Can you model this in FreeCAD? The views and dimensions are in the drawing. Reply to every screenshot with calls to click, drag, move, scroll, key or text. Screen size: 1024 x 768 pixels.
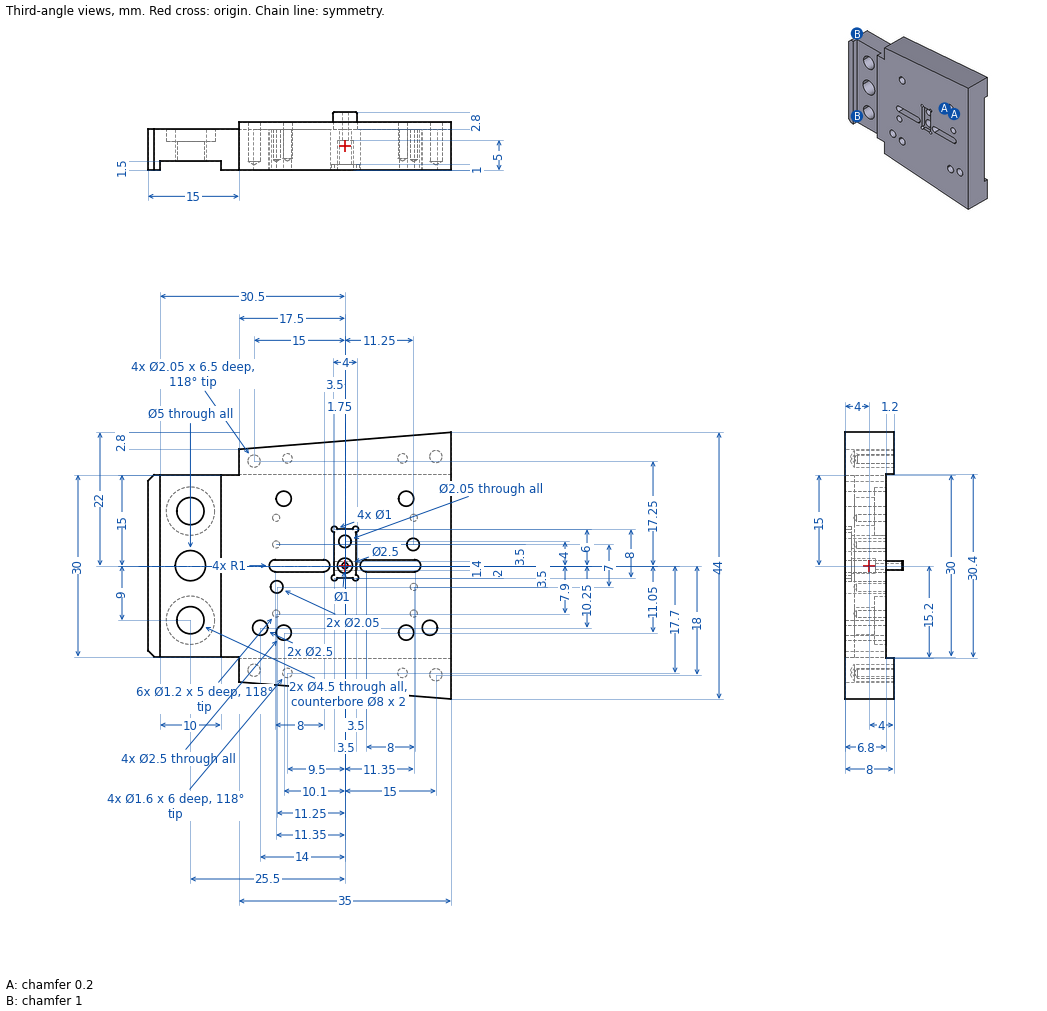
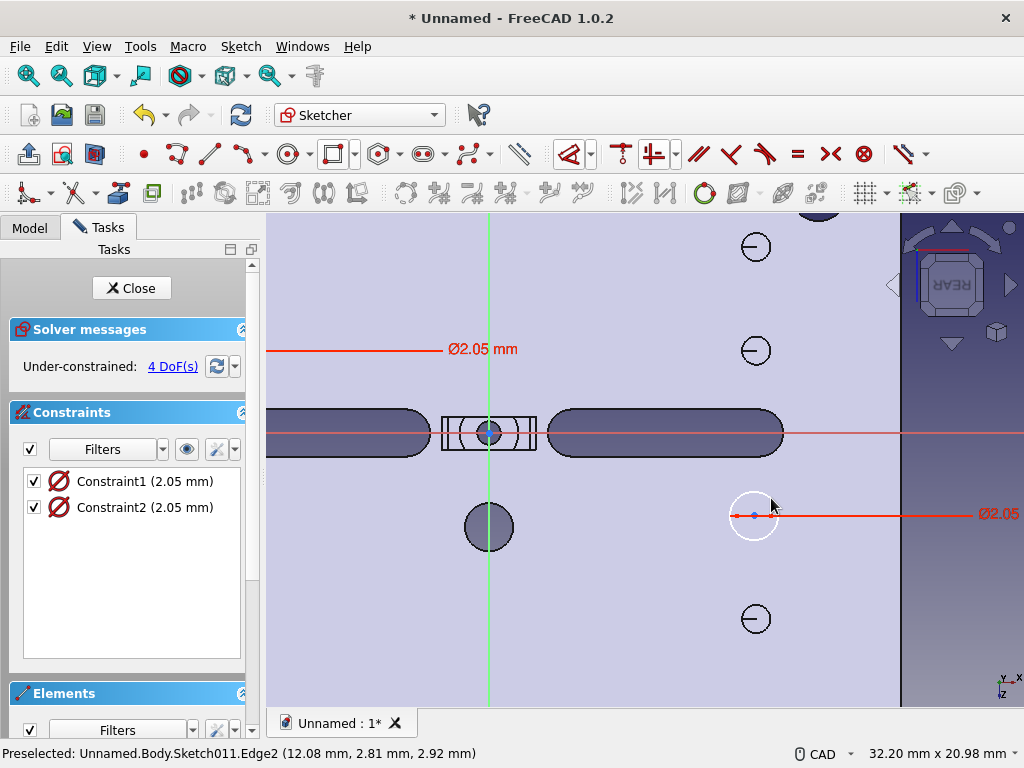
scroll(754, 515, down, 2)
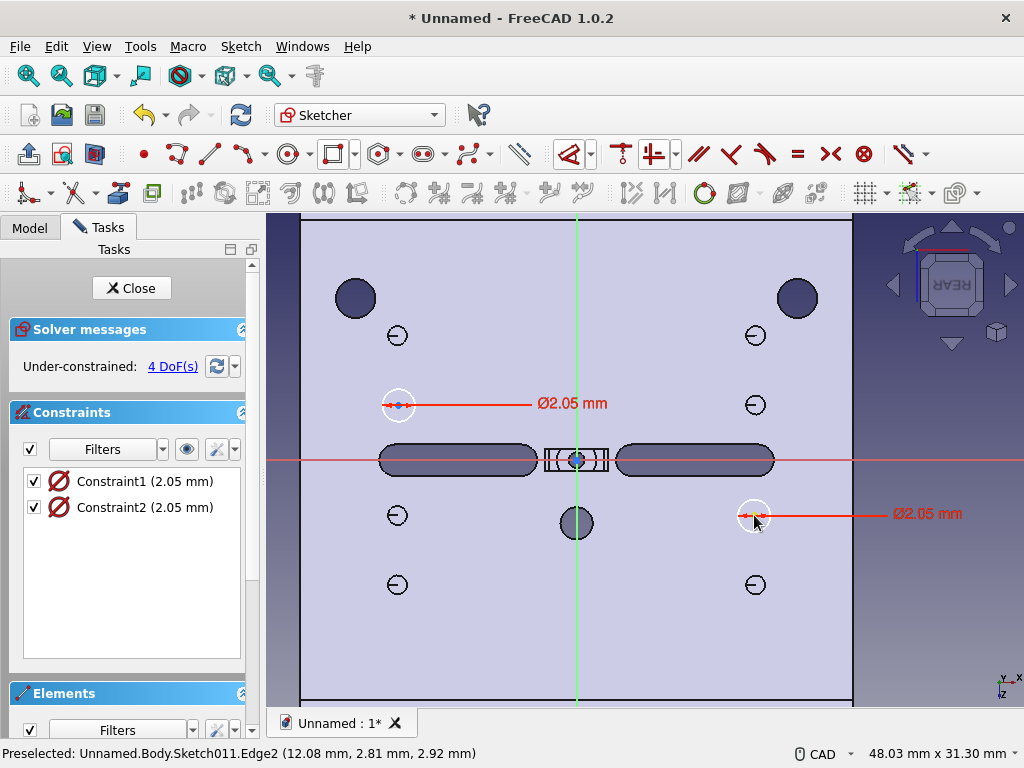
click(399, 405)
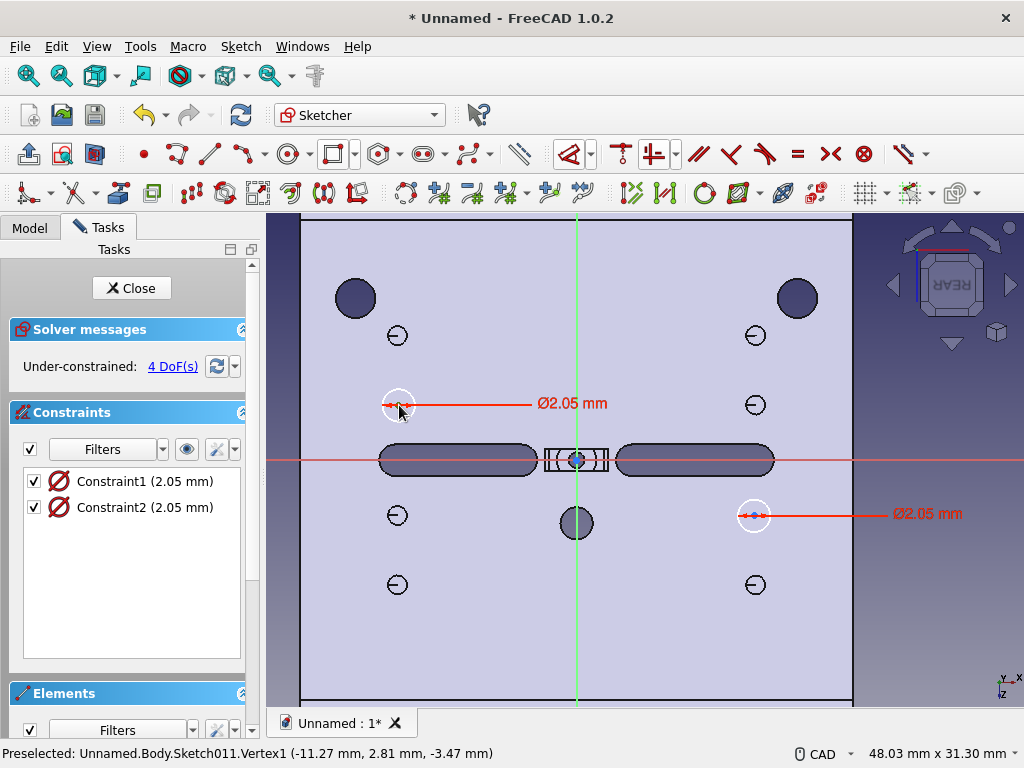
click(754, 516)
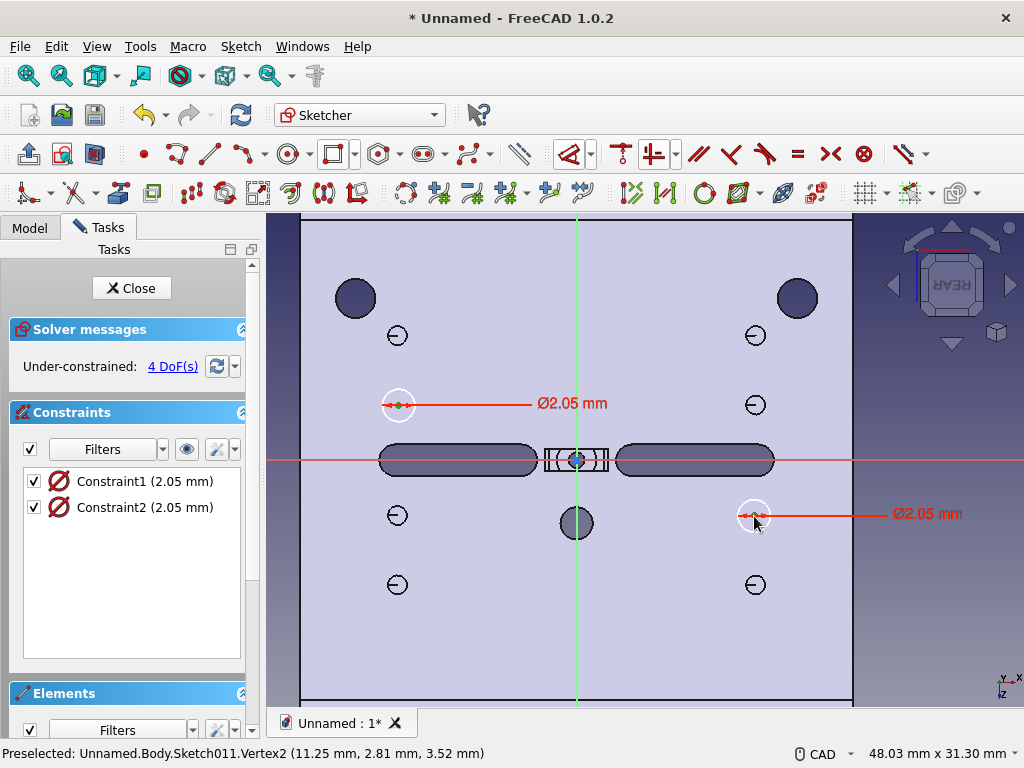
click(590, 154)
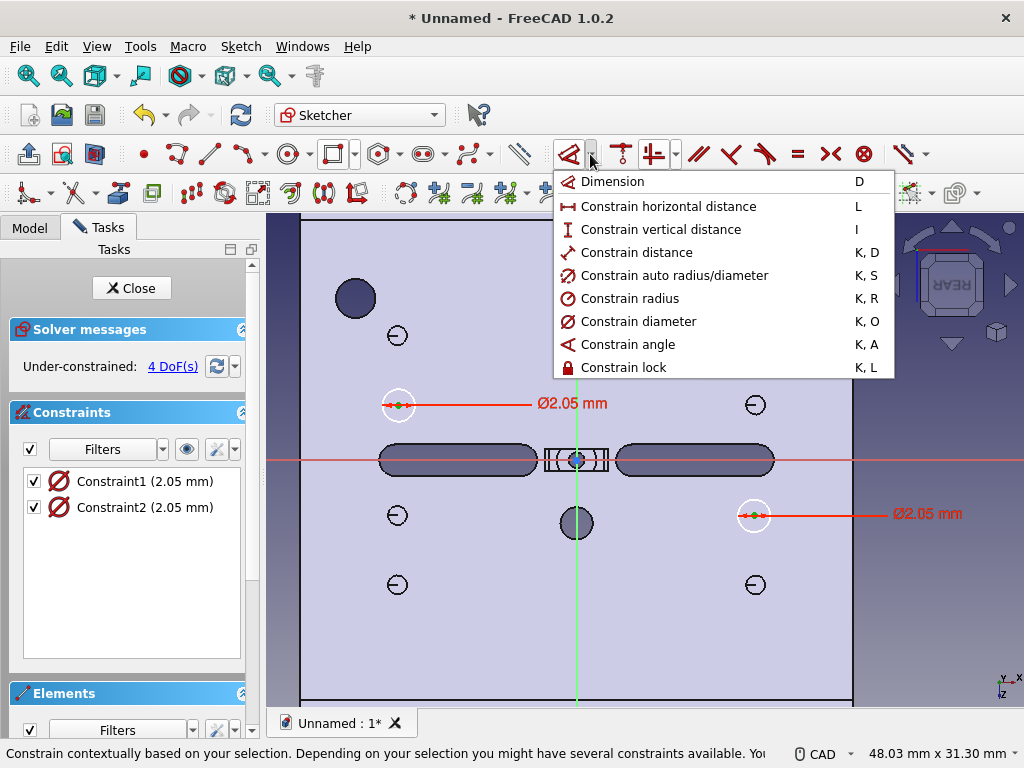
click(724, 230)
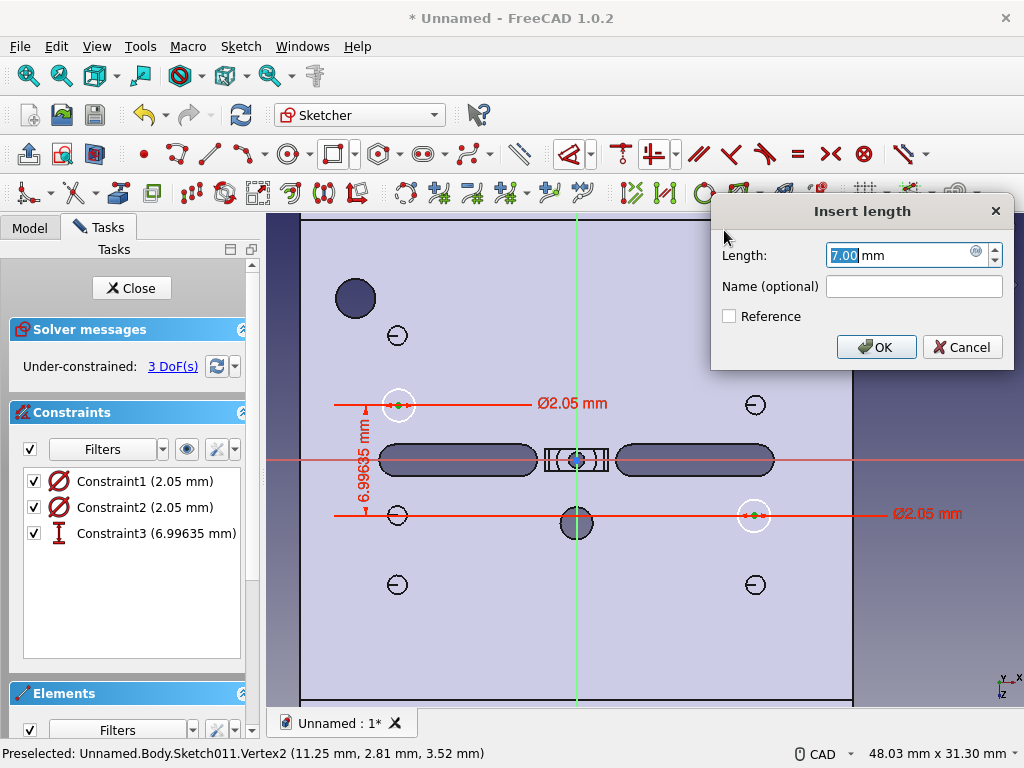
text(7)
key(Return)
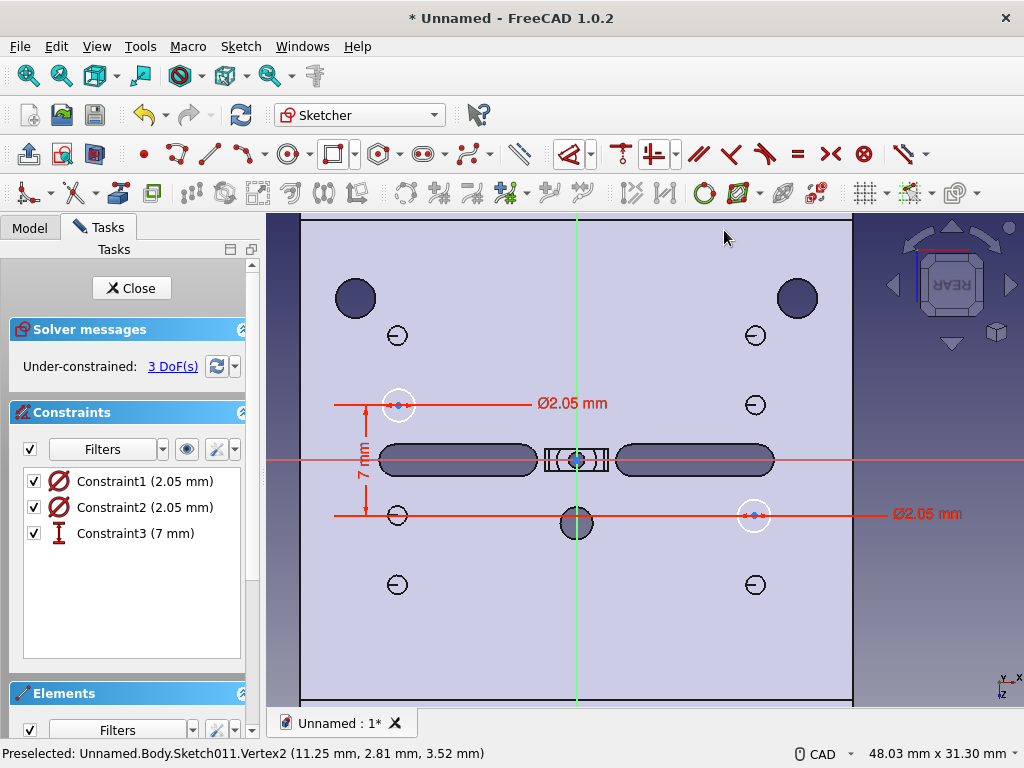
click(399, 405)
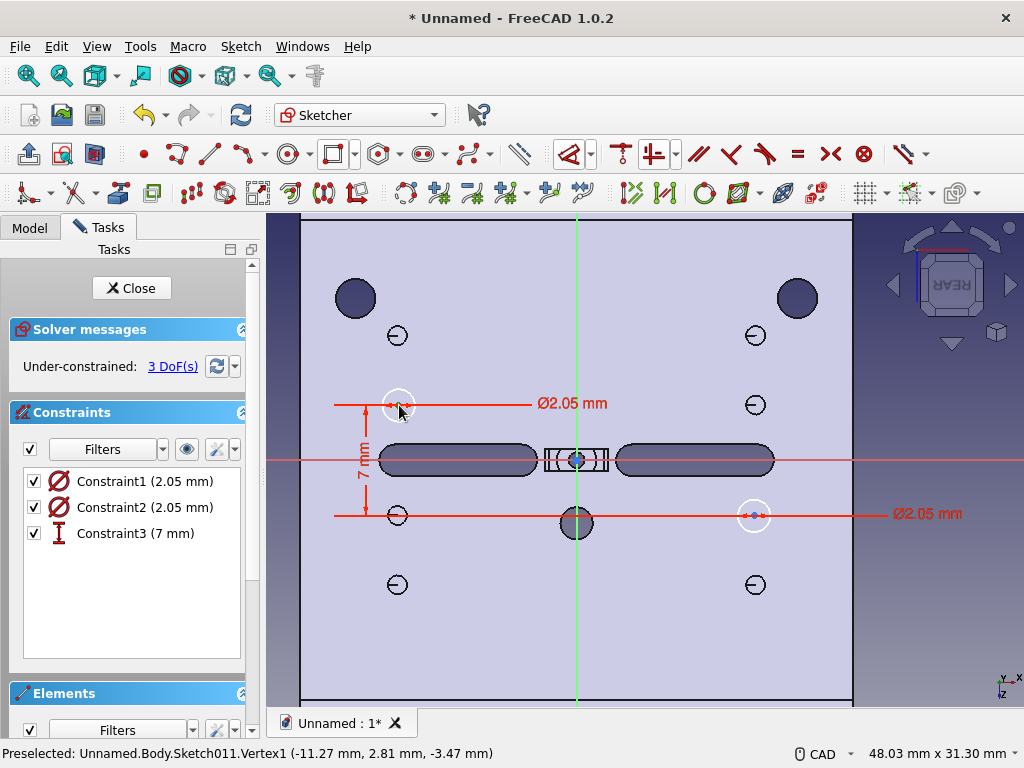
key(i)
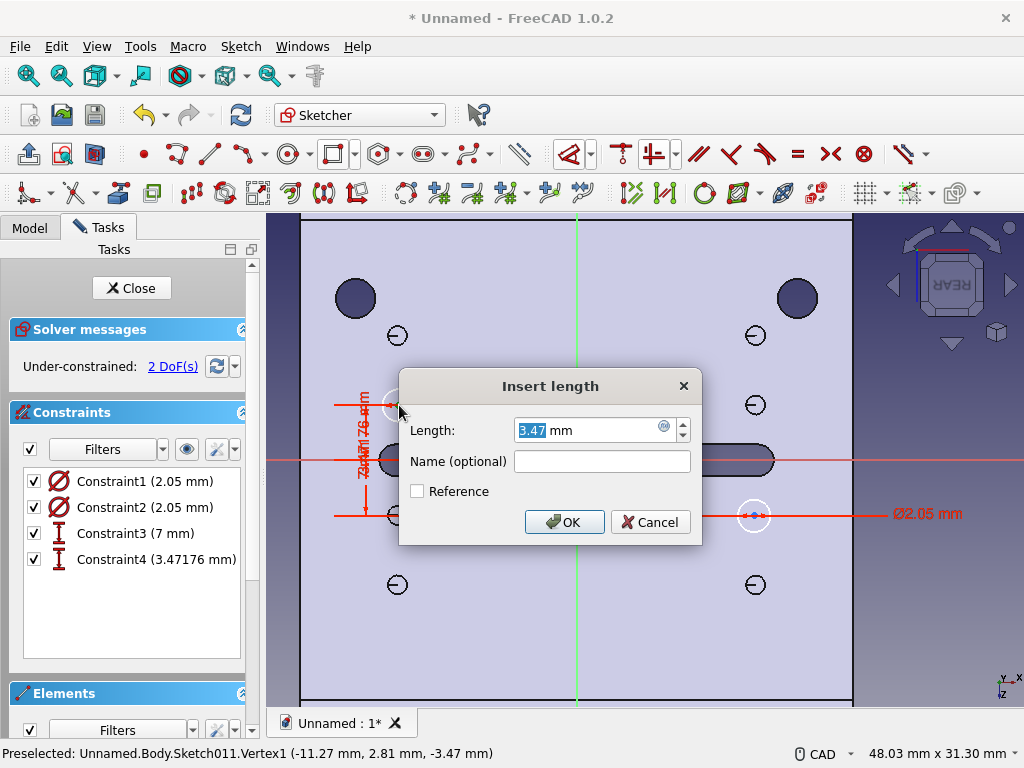
text(3.5)
key(Return)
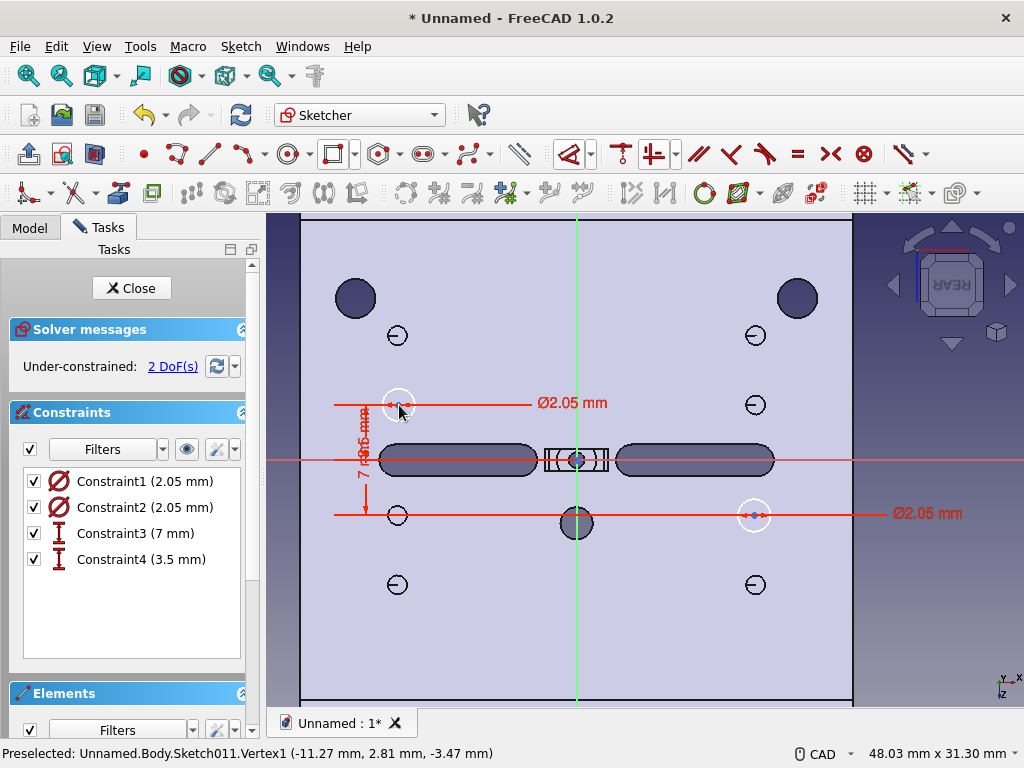
click(399, 405)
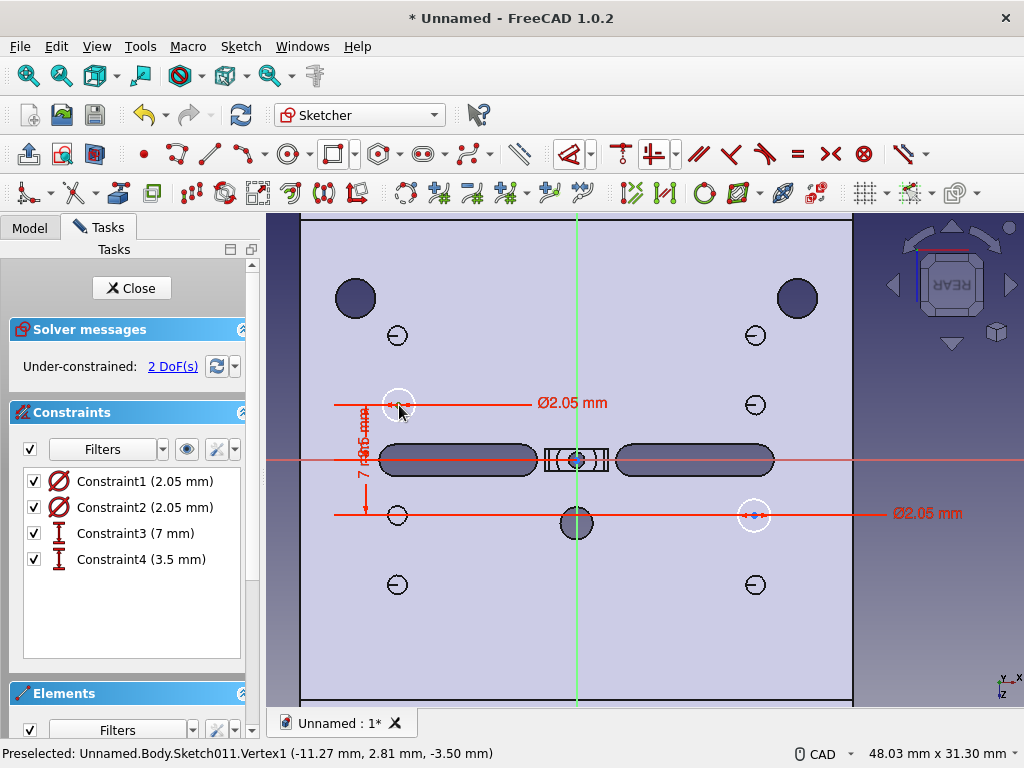
key(l)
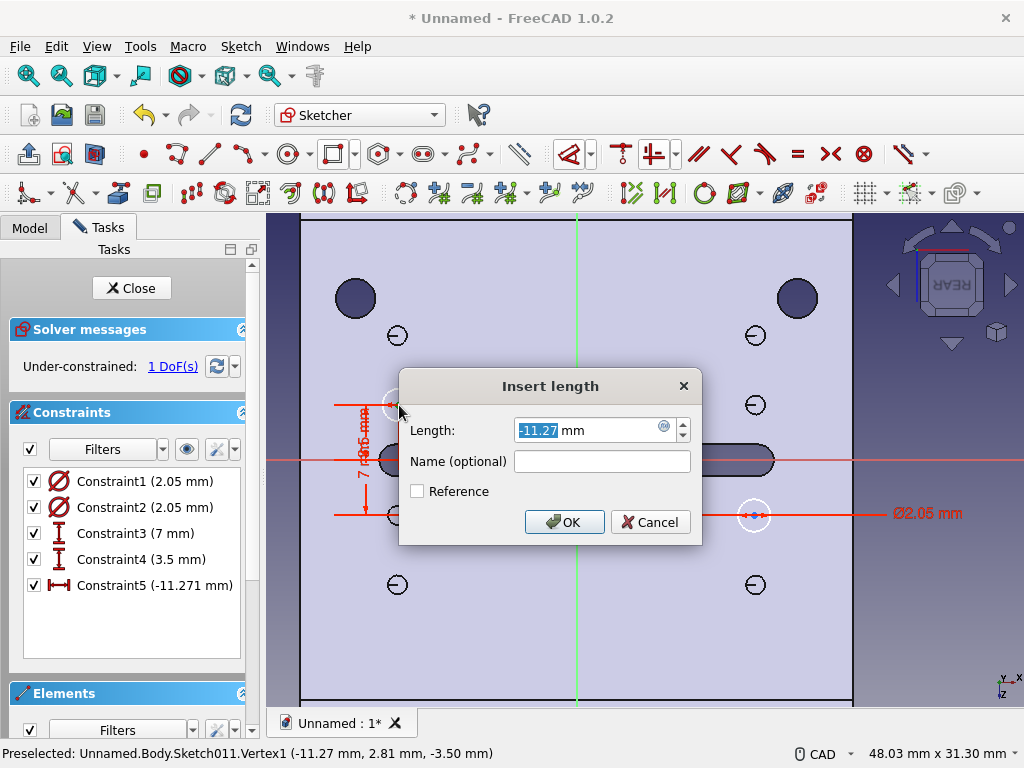
text(-11.25)
key(Return)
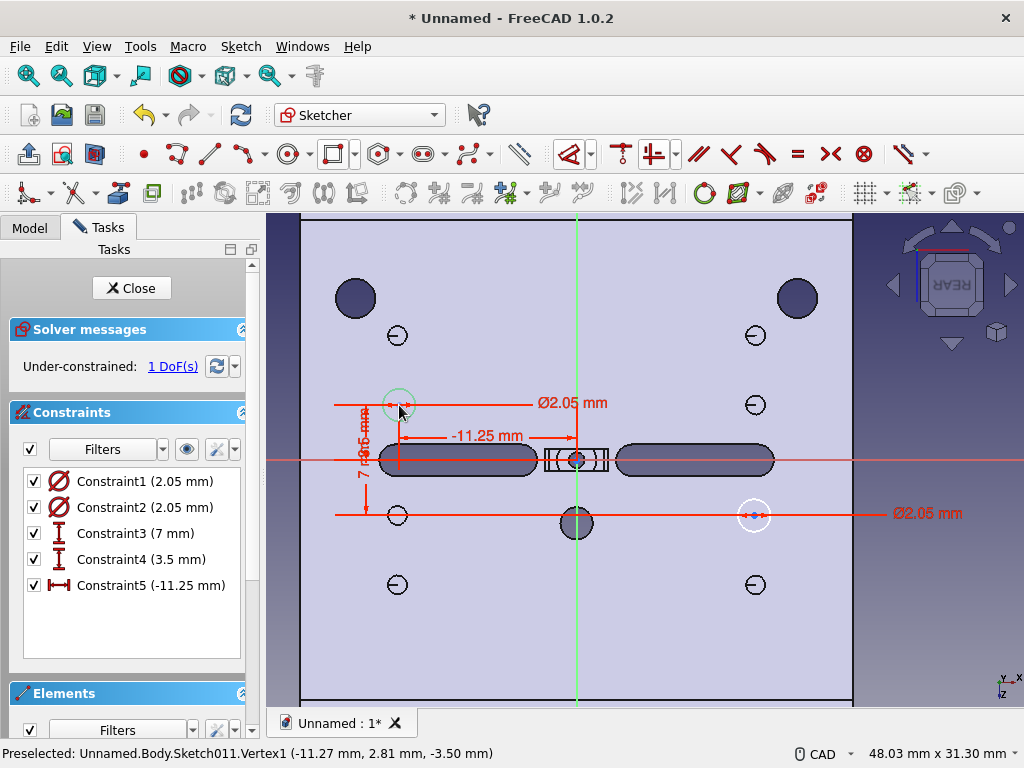
click(754, 515)